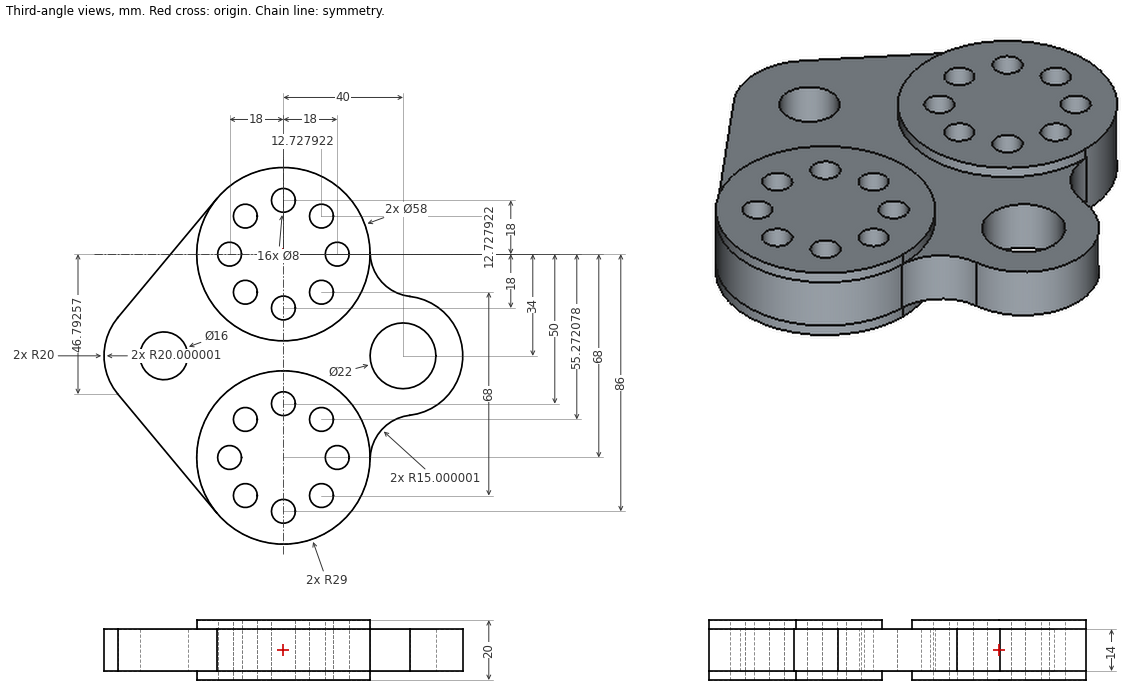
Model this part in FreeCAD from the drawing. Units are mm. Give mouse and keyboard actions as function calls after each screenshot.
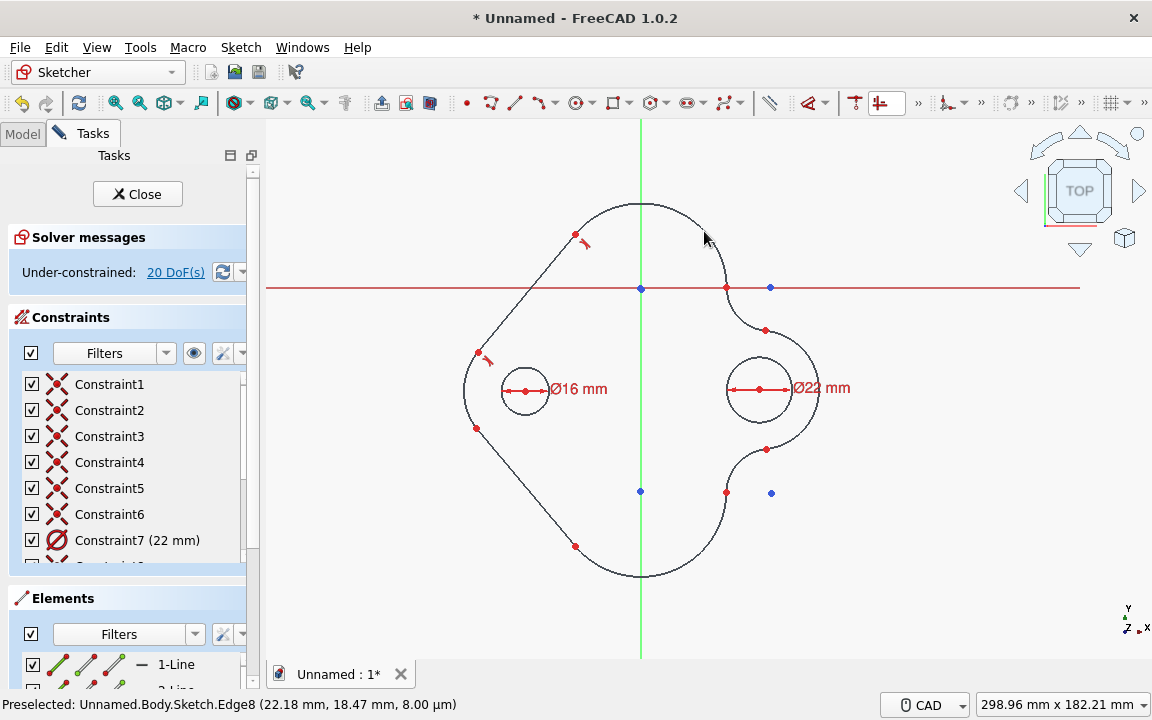
click(506, 463)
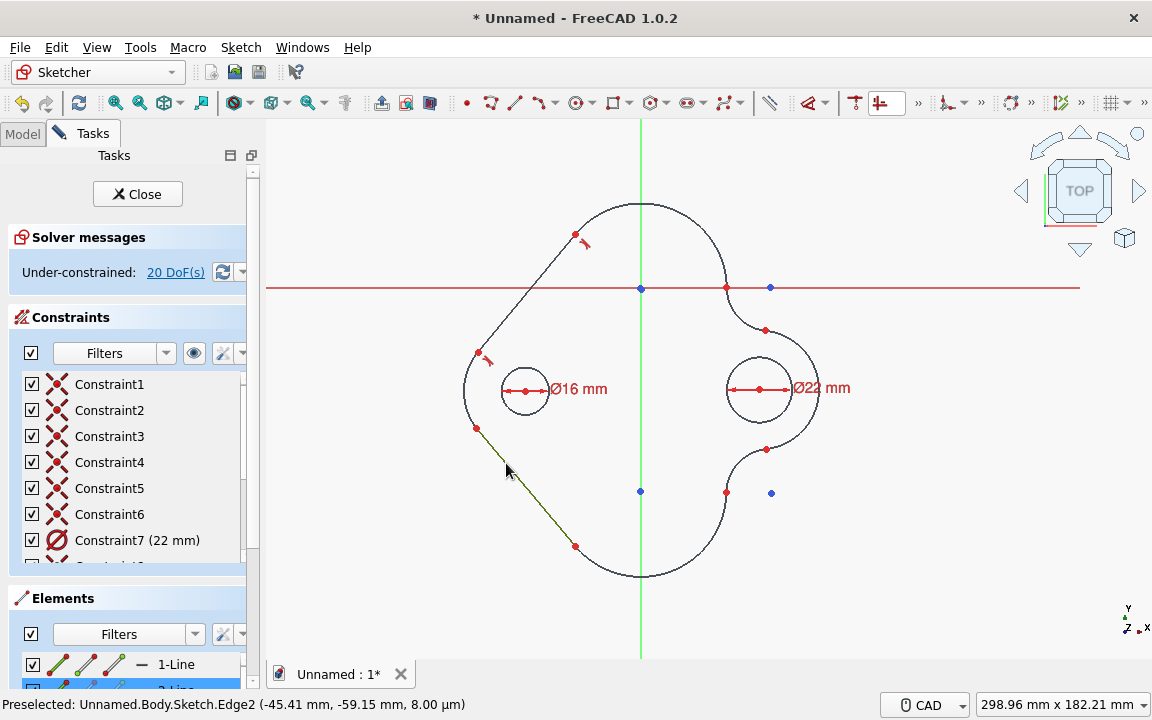
click(467, 374)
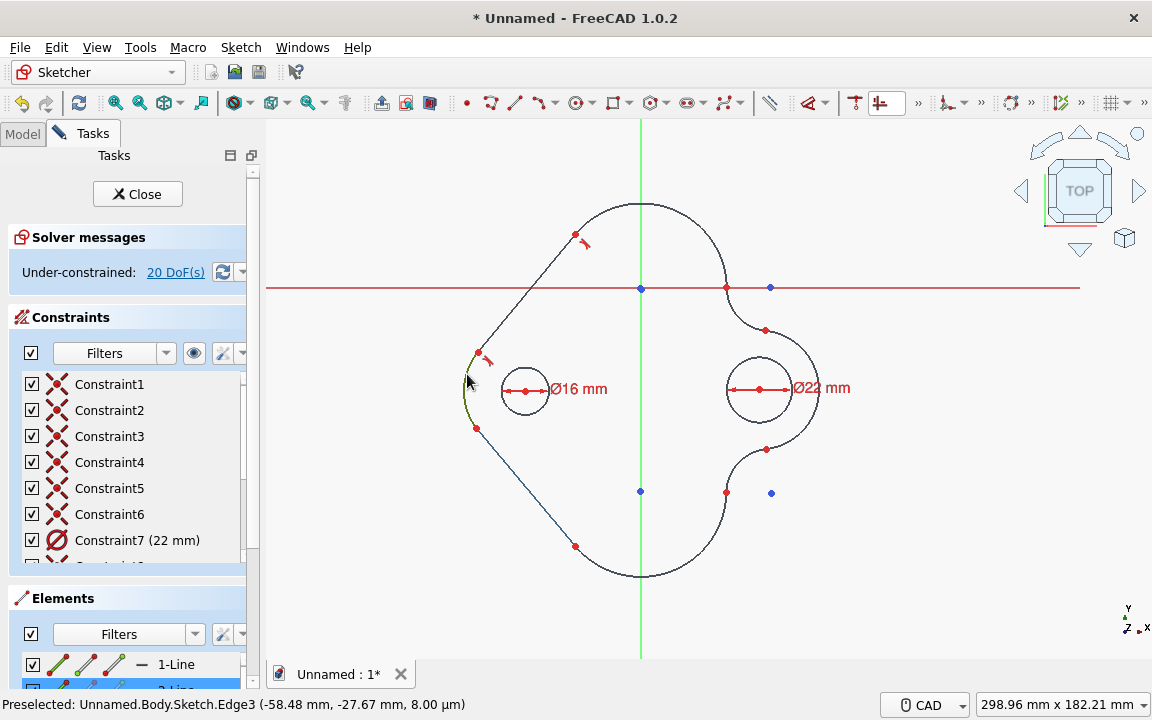
key(t)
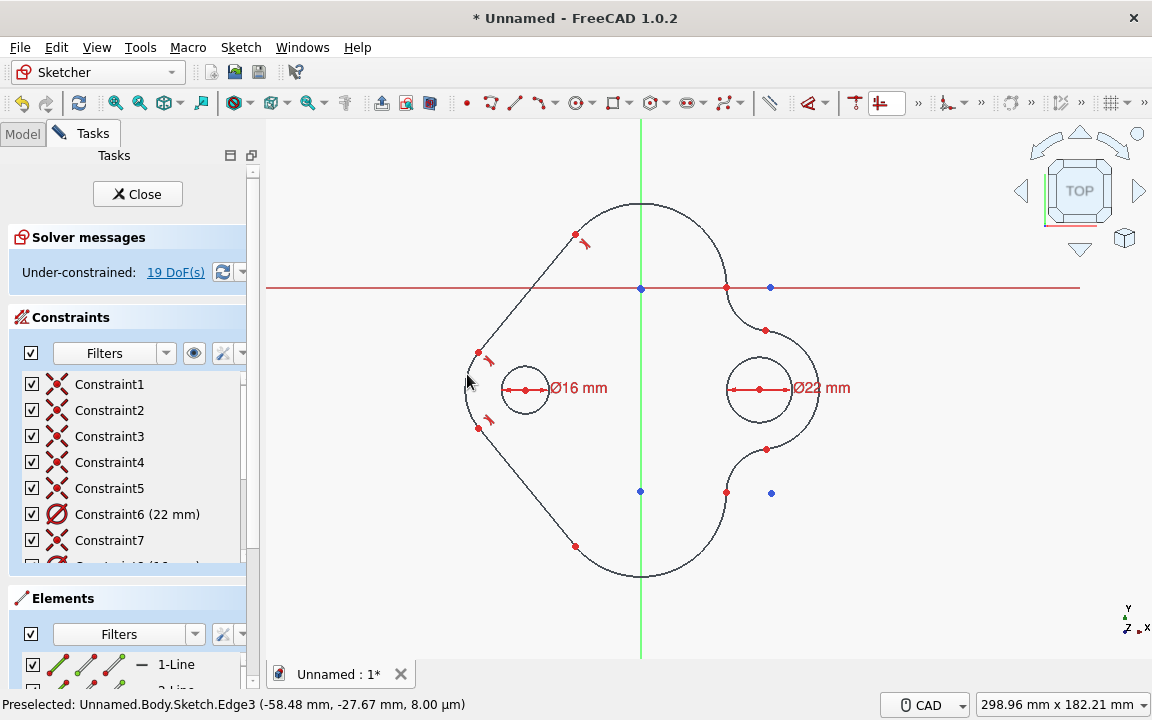
click(508, 463)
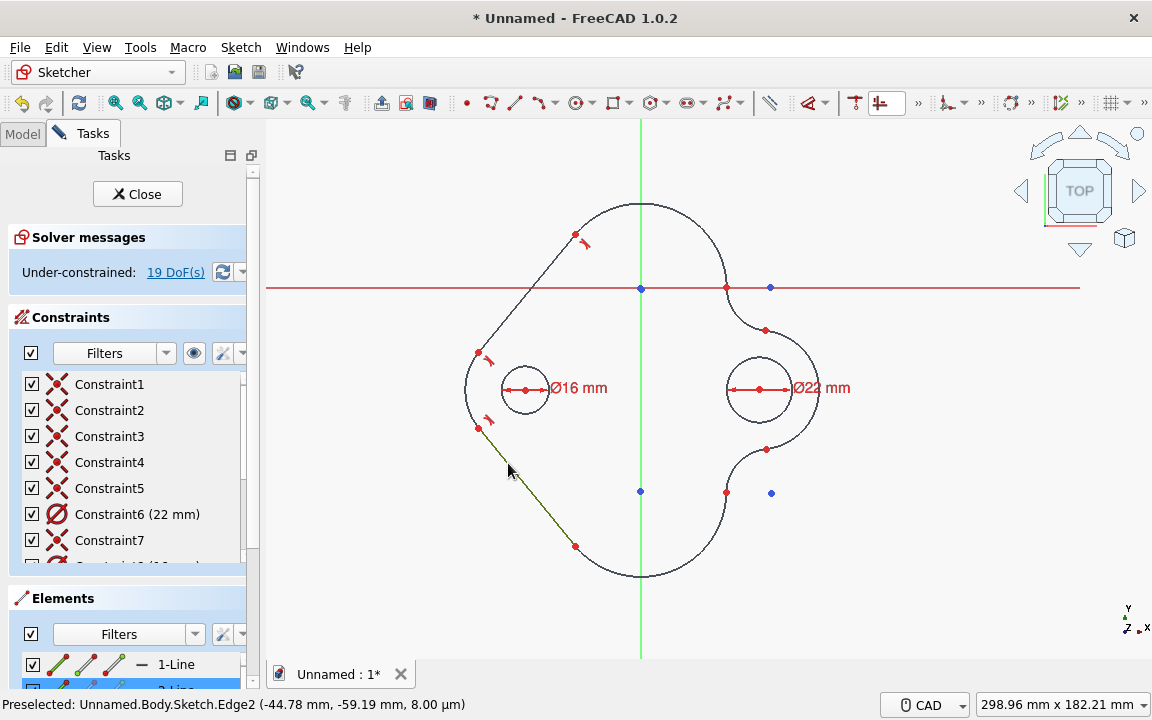
click(629, 576)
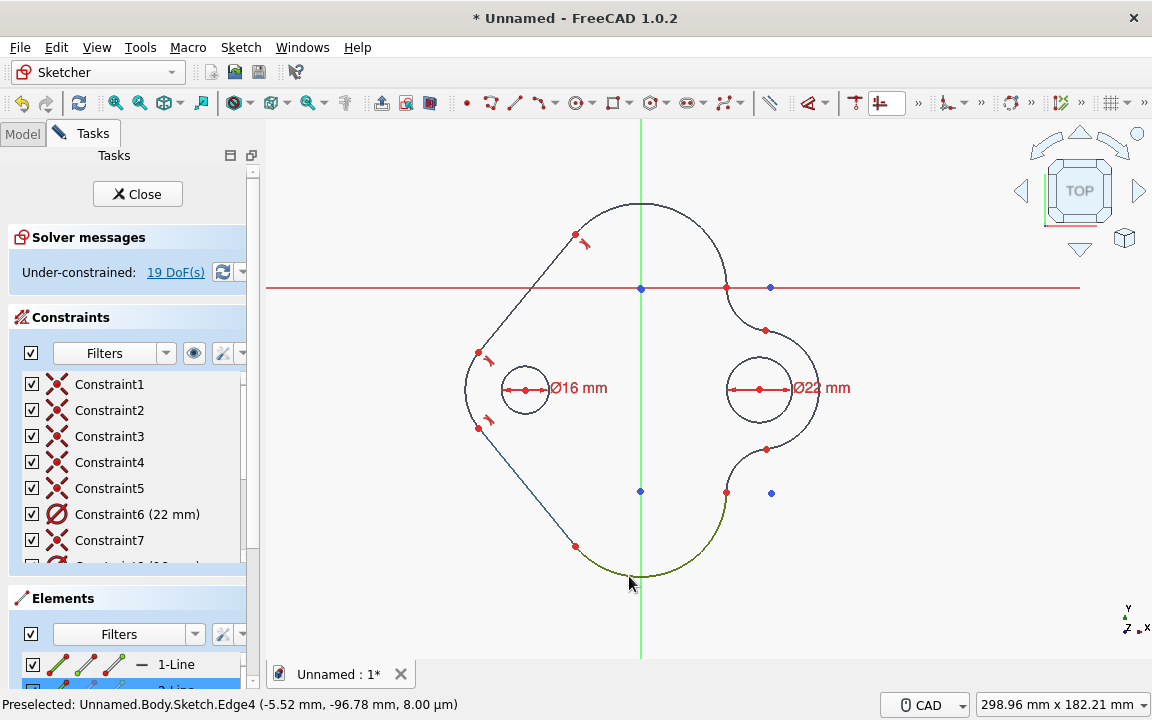
key(t)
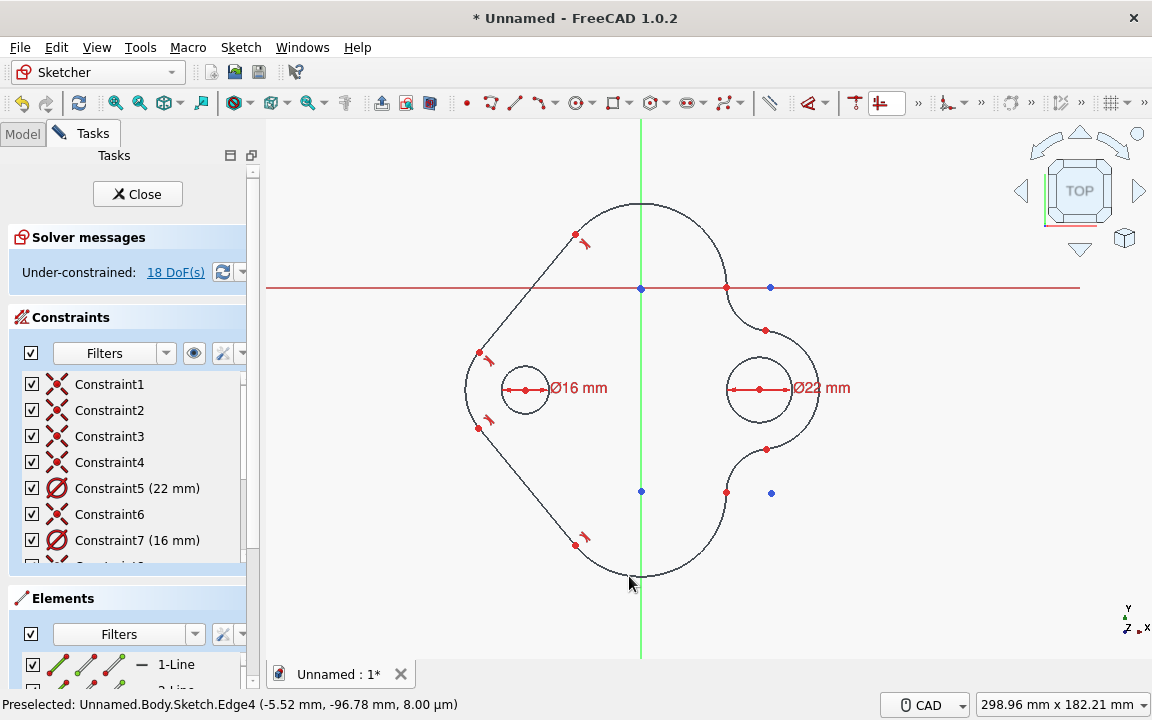
click(628, 576)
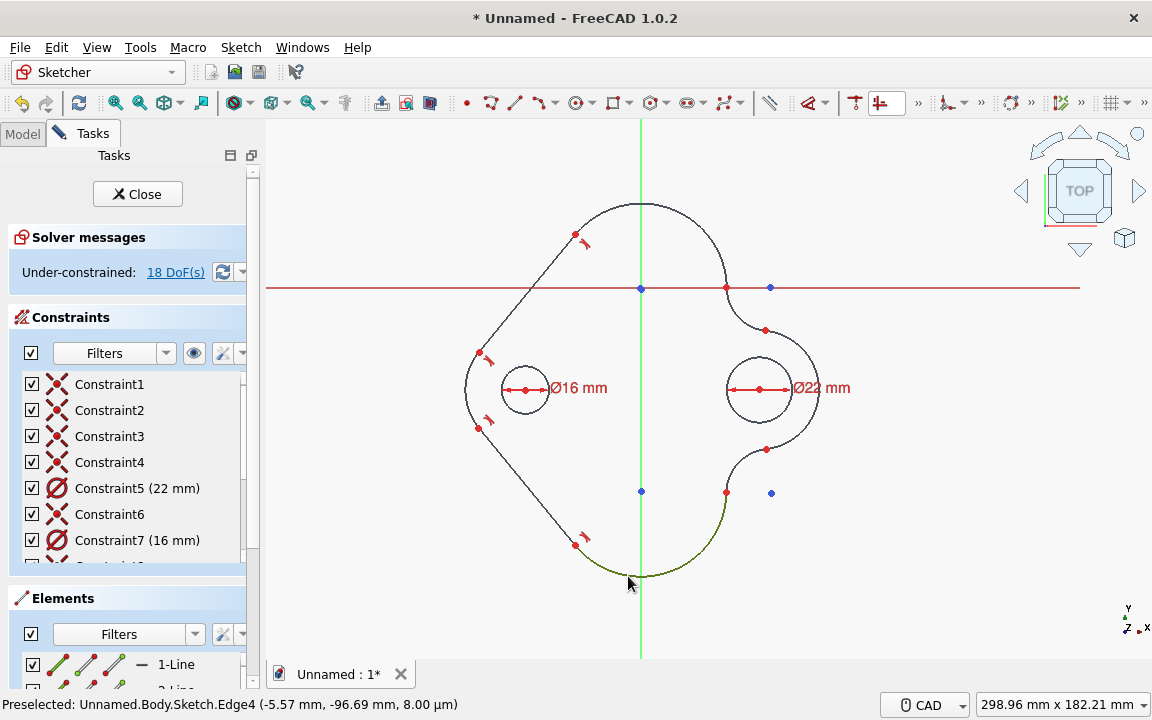
click(748, 455)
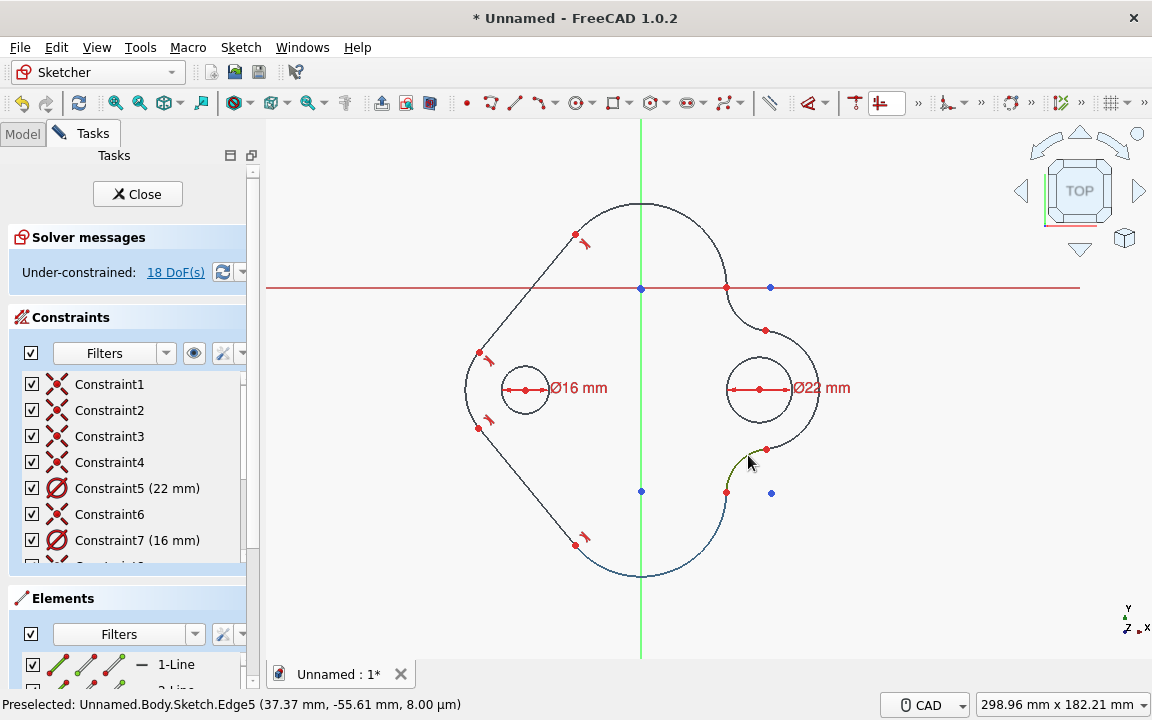
key(t)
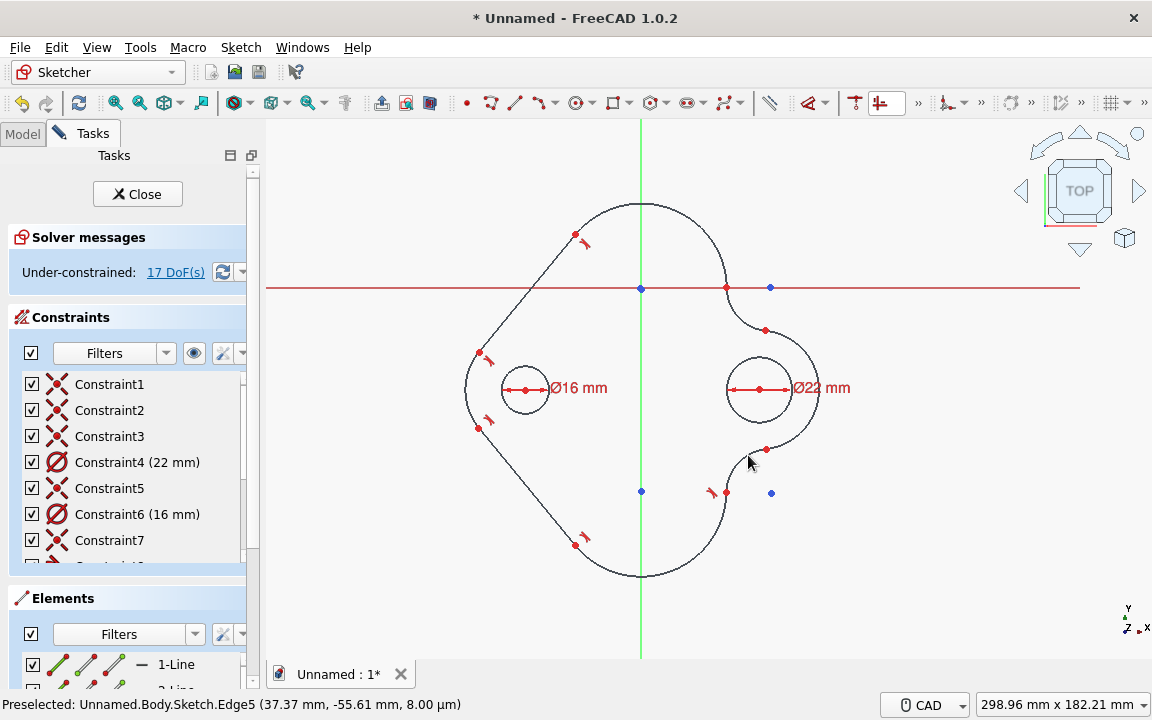
click(748, 455)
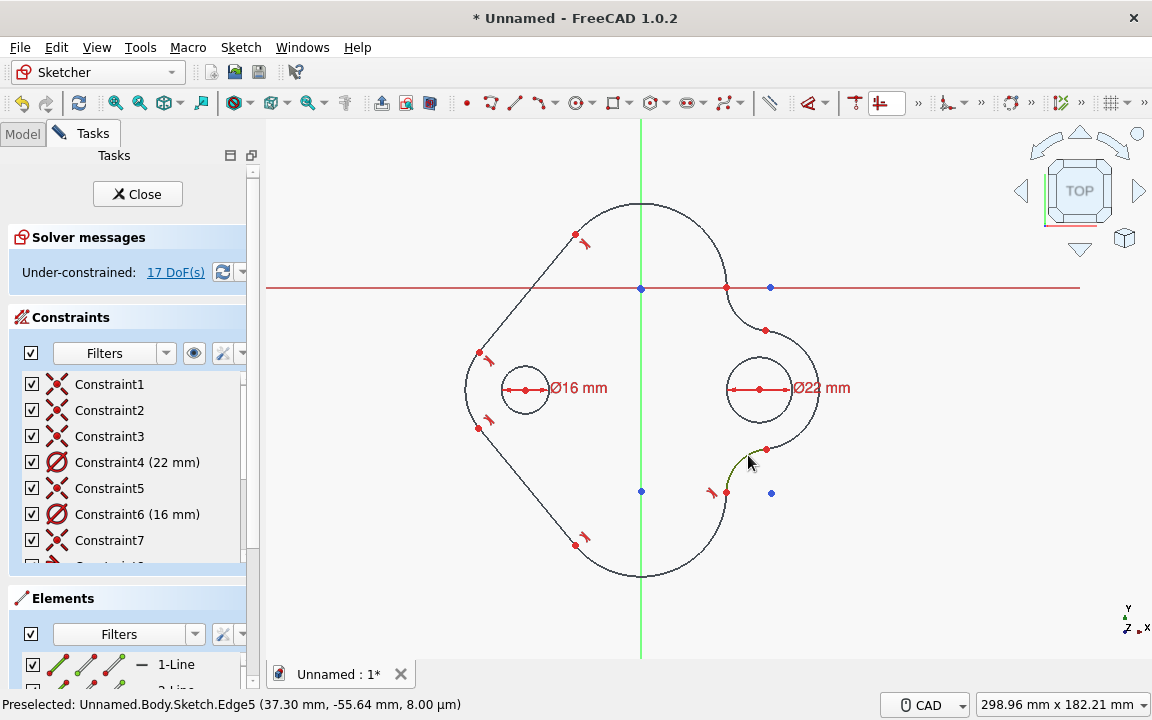
click(809, 423)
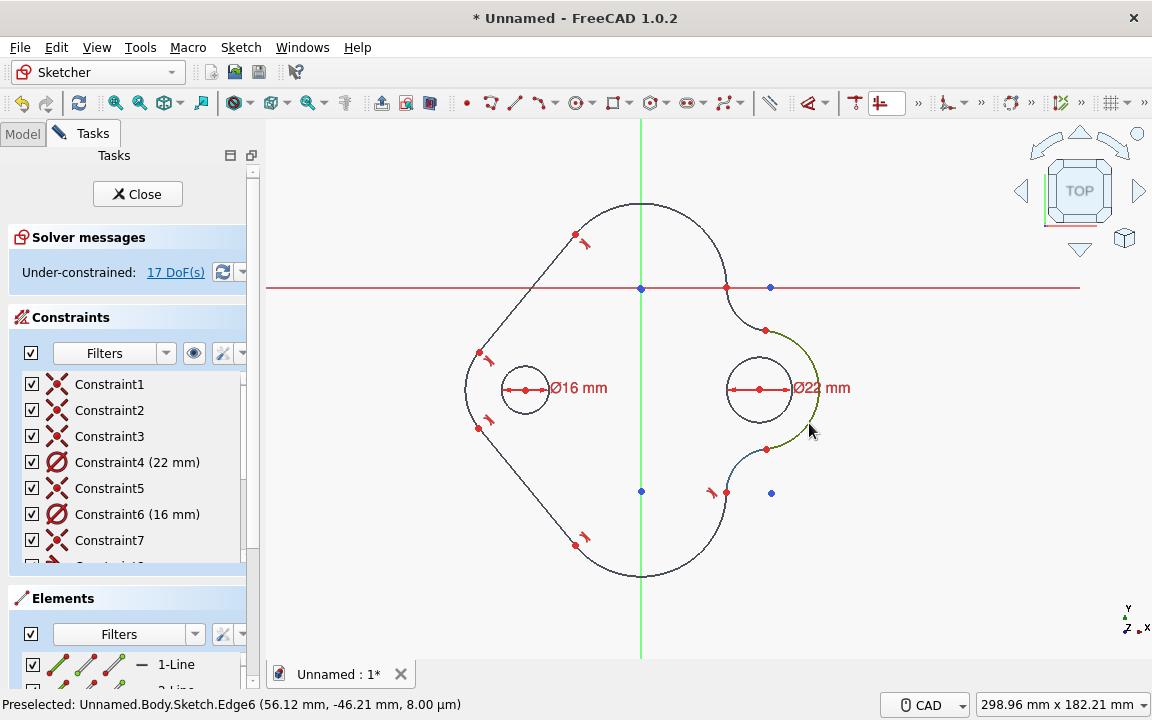
key(t)